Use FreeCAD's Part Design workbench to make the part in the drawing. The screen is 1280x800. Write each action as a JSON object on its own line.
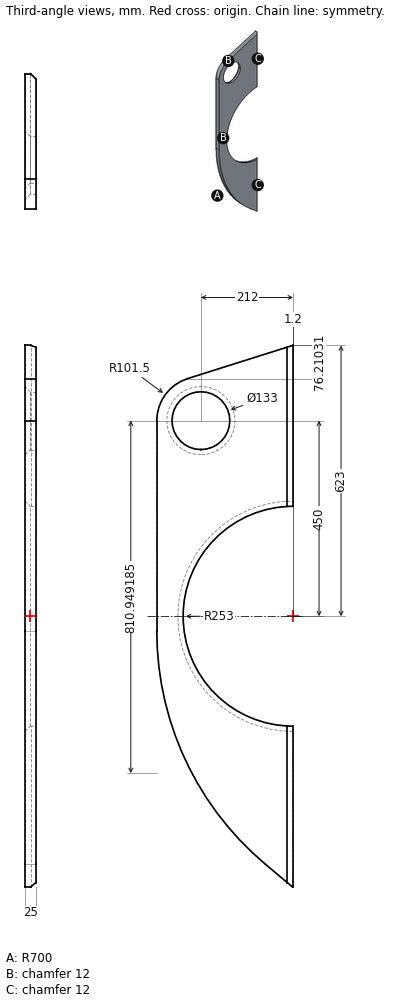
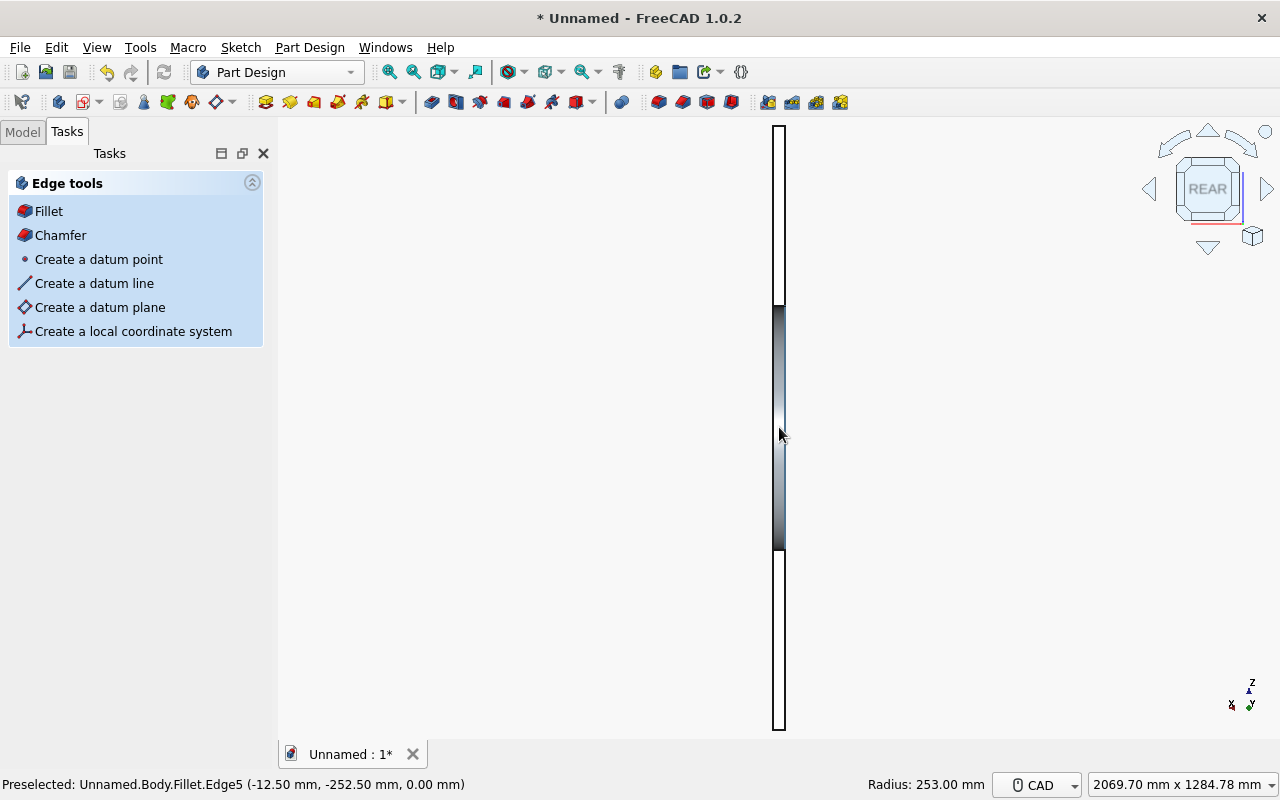
{"action": "key", "text": "6"}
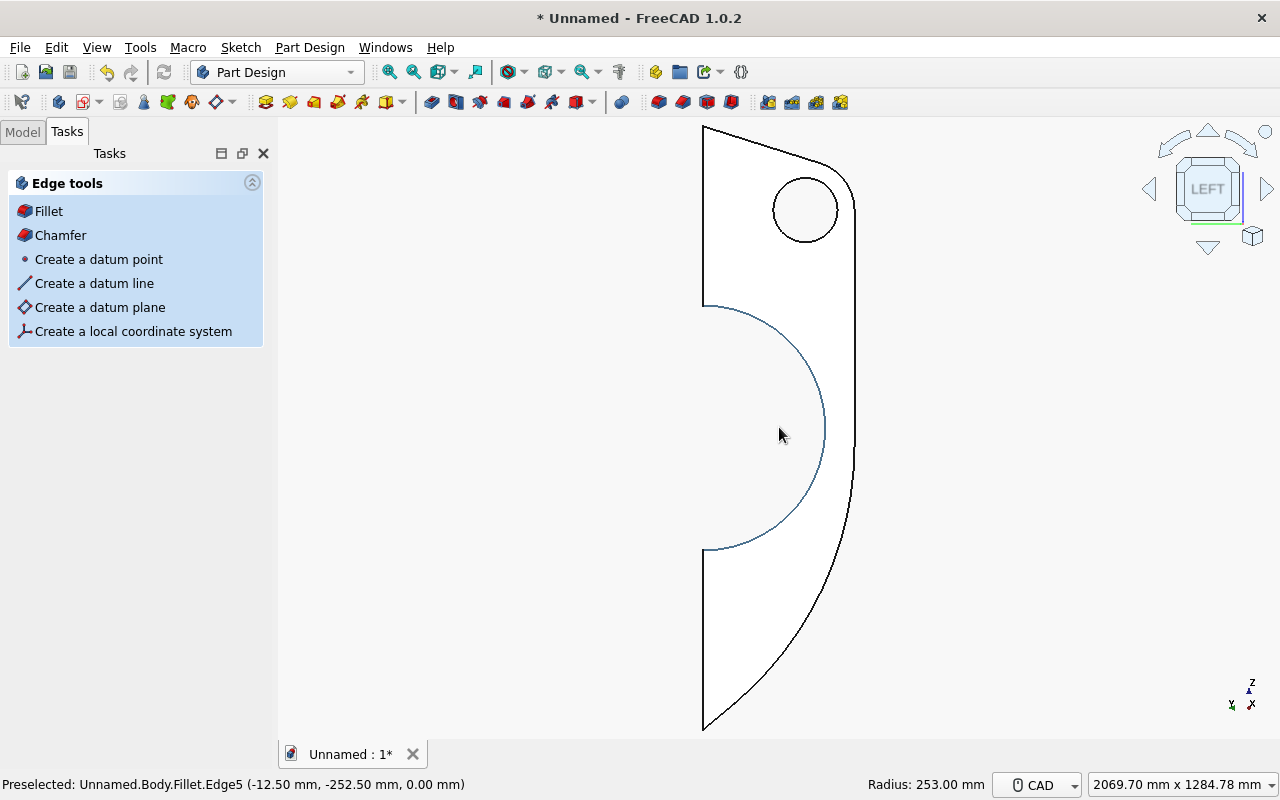
{"action": "left_click", "coordinate": [838, 209], "text": "ctrl"}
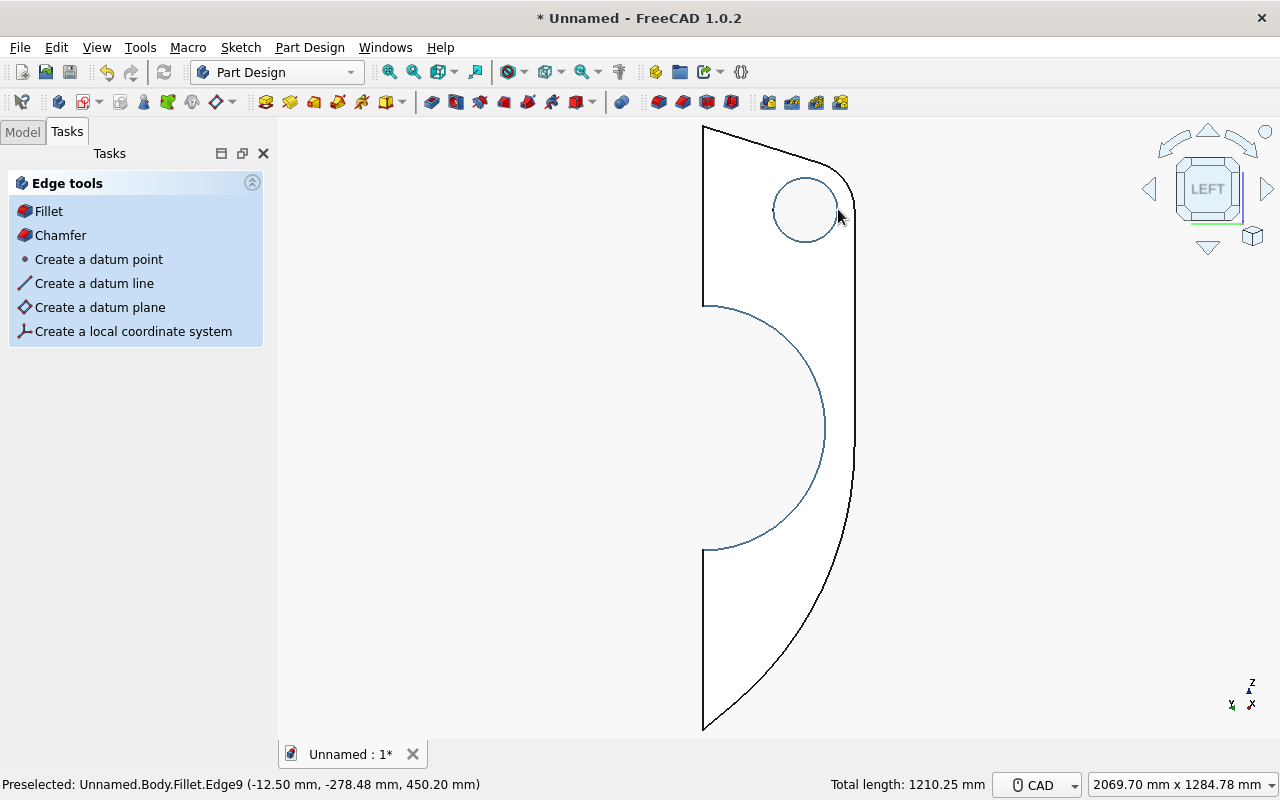
{"action": "left_click", "coordinate": [684, 102]}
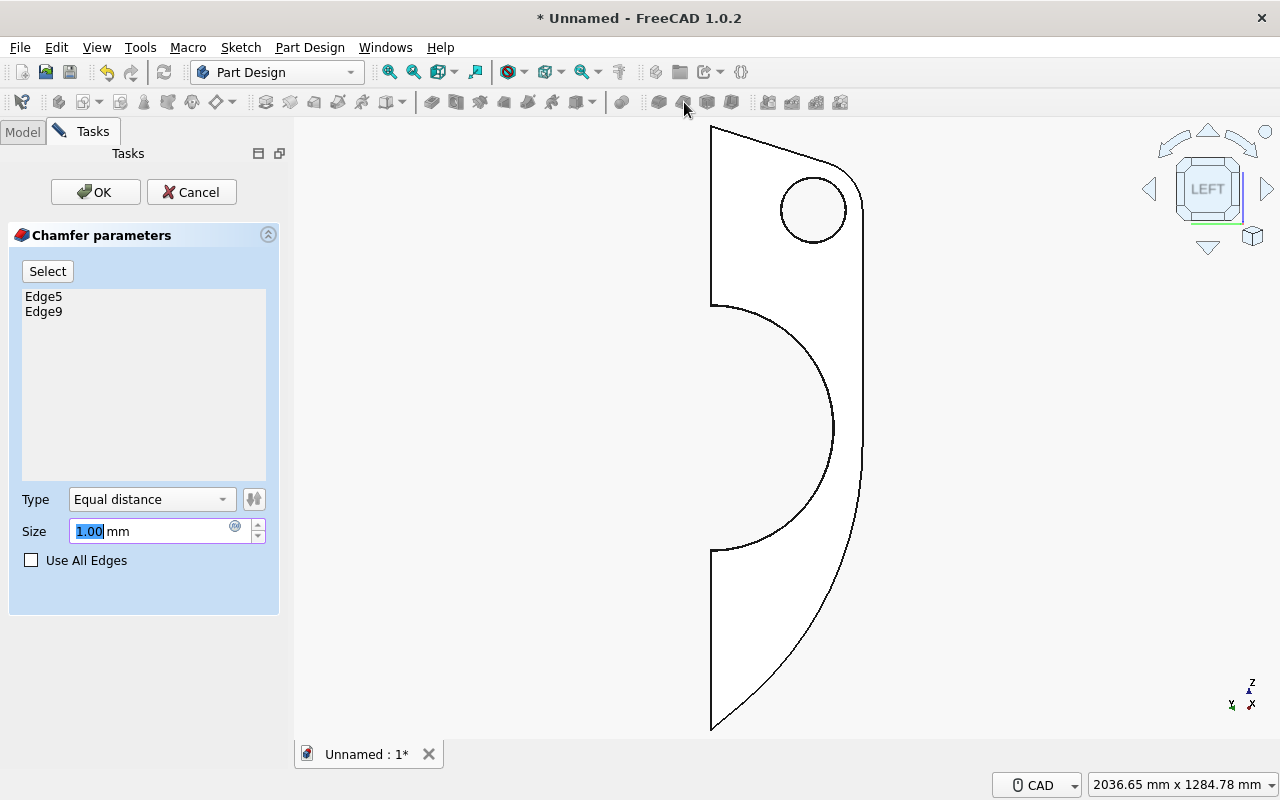
{"action": "type", "text": "12"}
{"action": "key", "text": "Tab"}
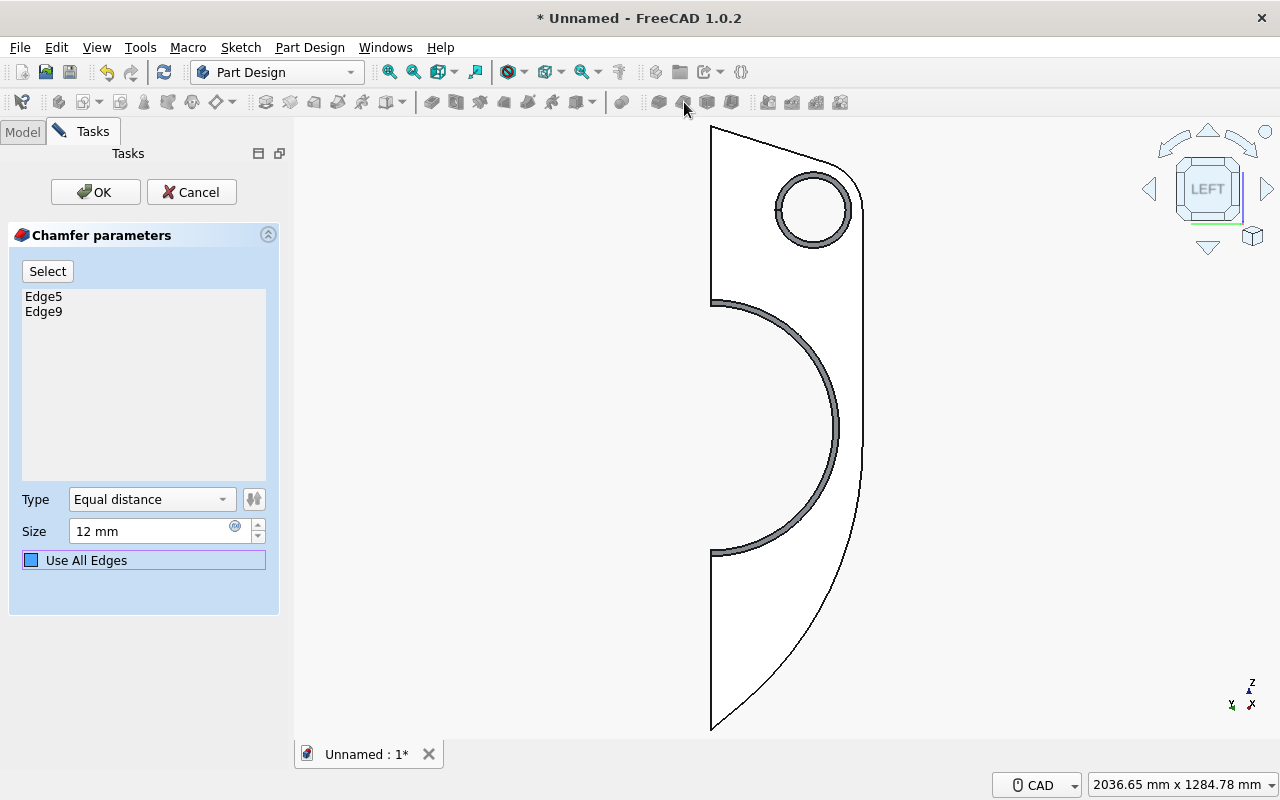
{"action": "left_click", "coordinate": [96, 192]}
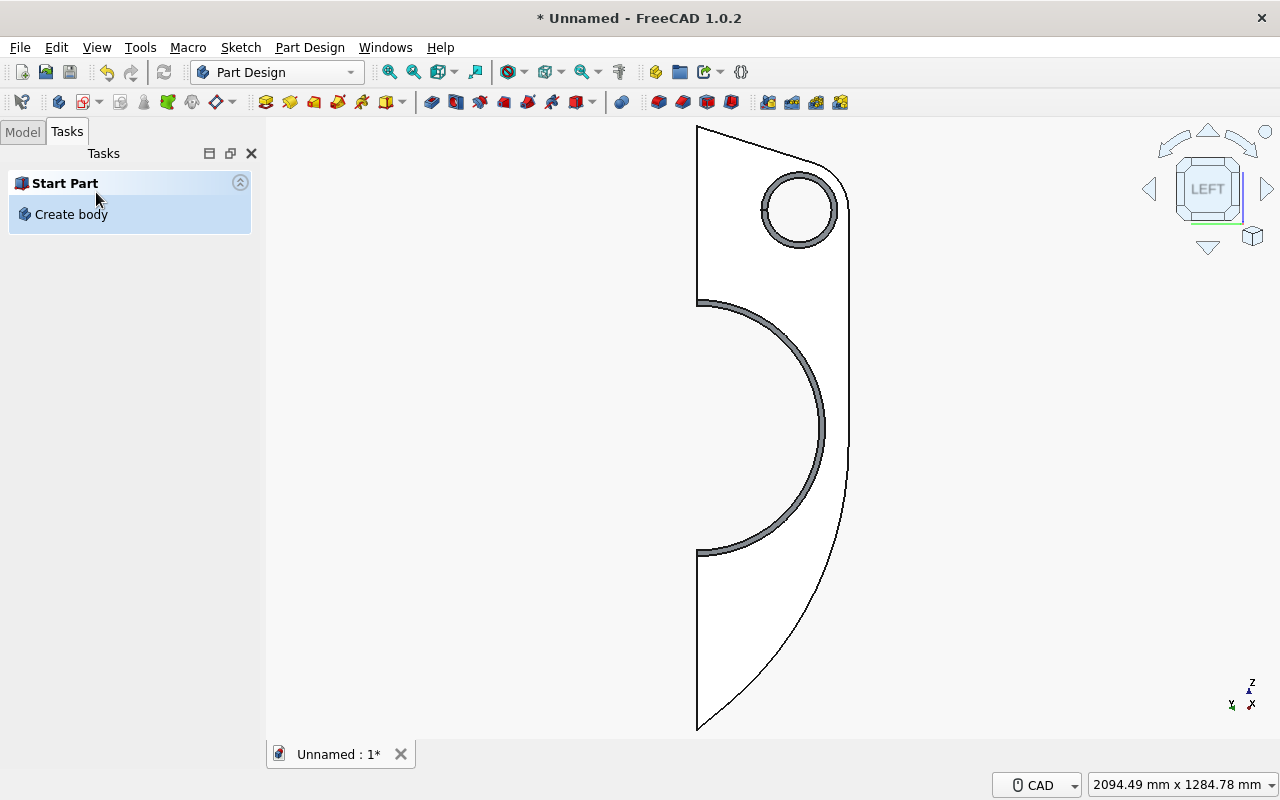
{"action": "key", "text": "0"}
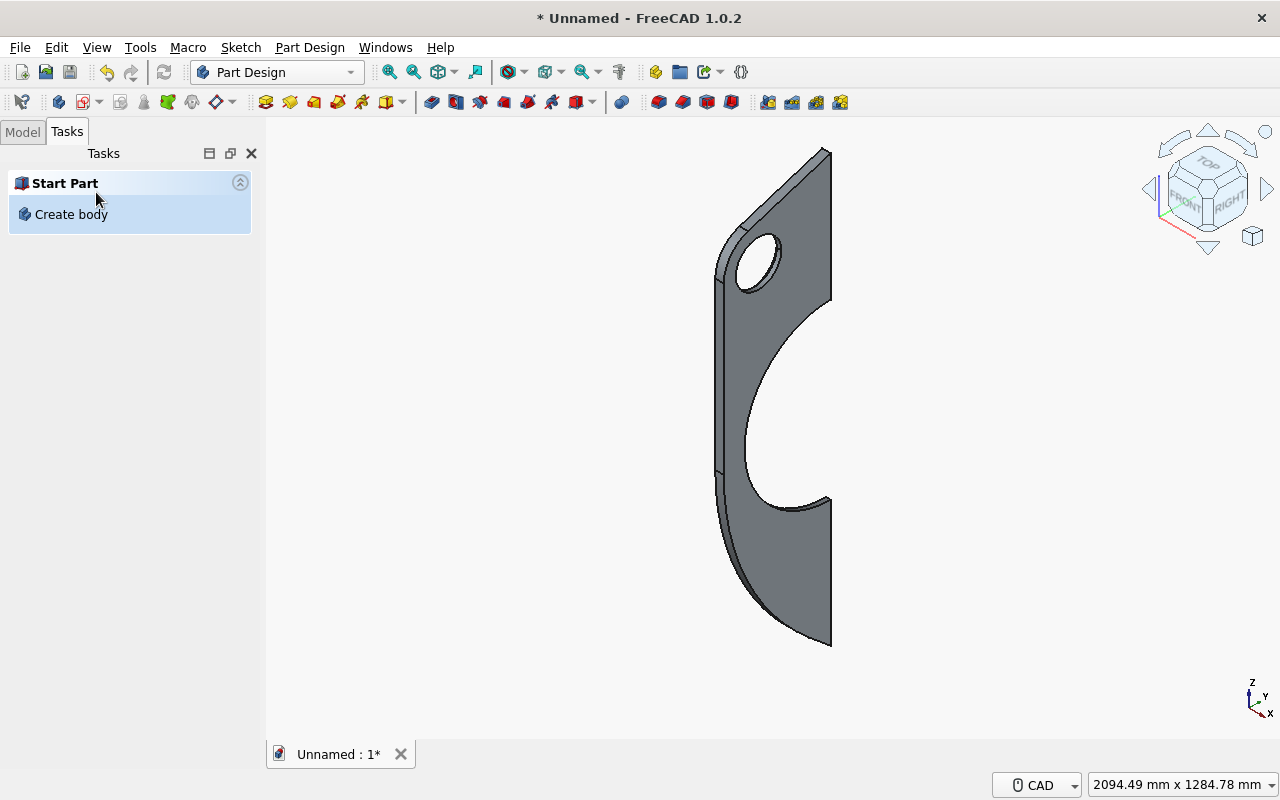
{"action": "key", "text": "2"}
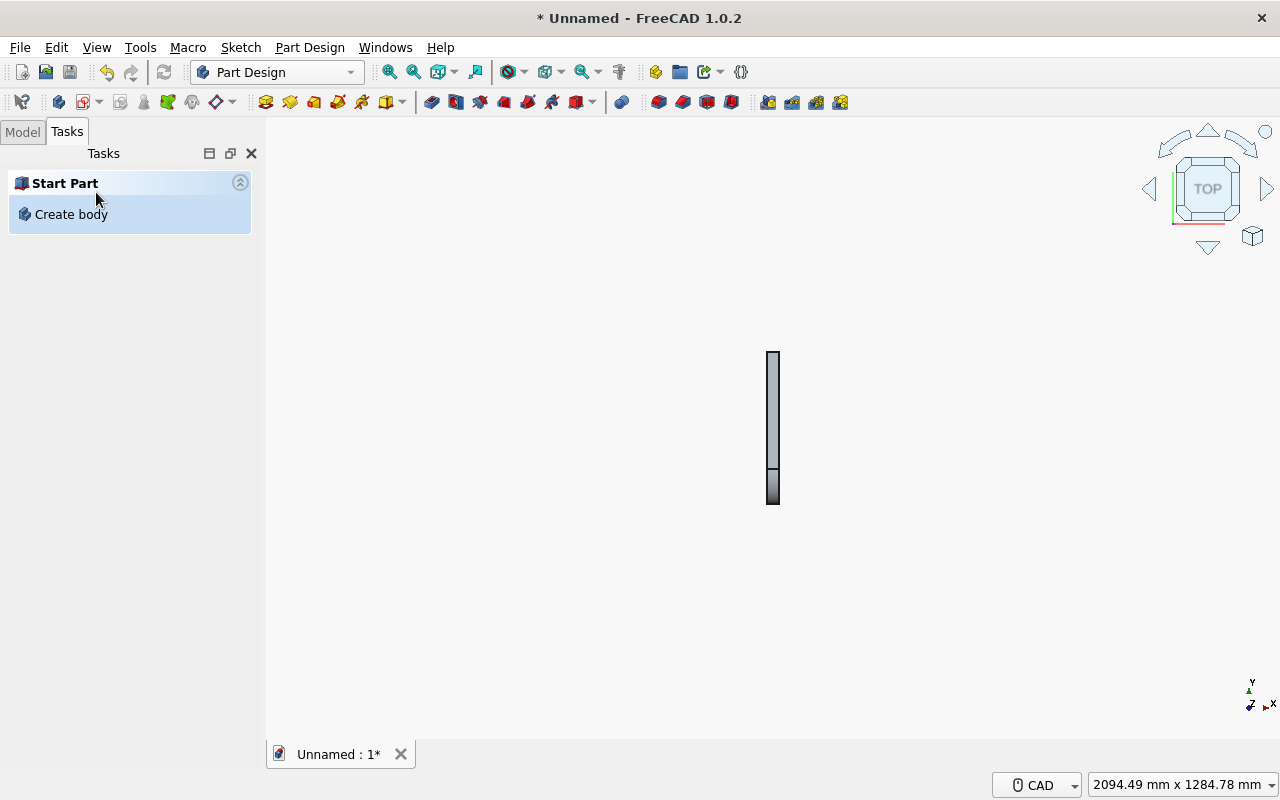
{"action": "left_click", "coordinate": [390, 72]}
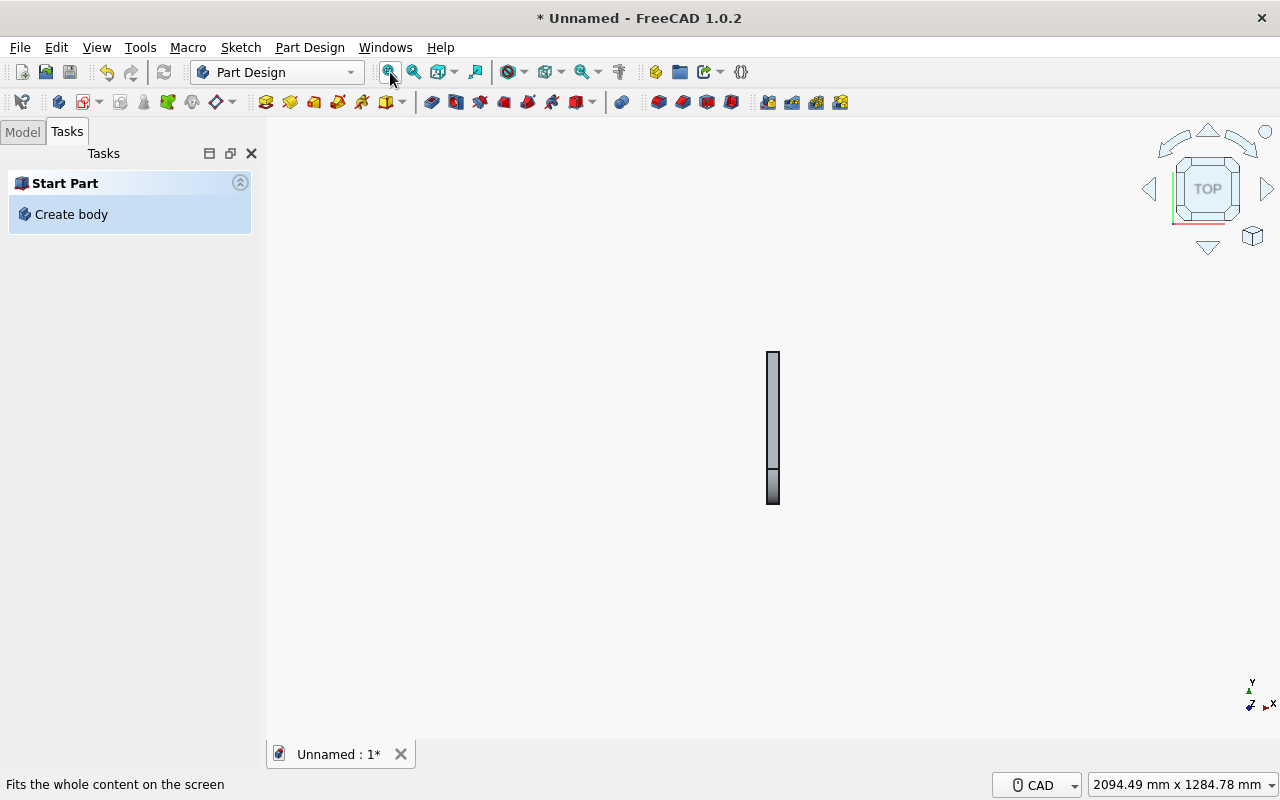
{"action": "key", "text": "1"}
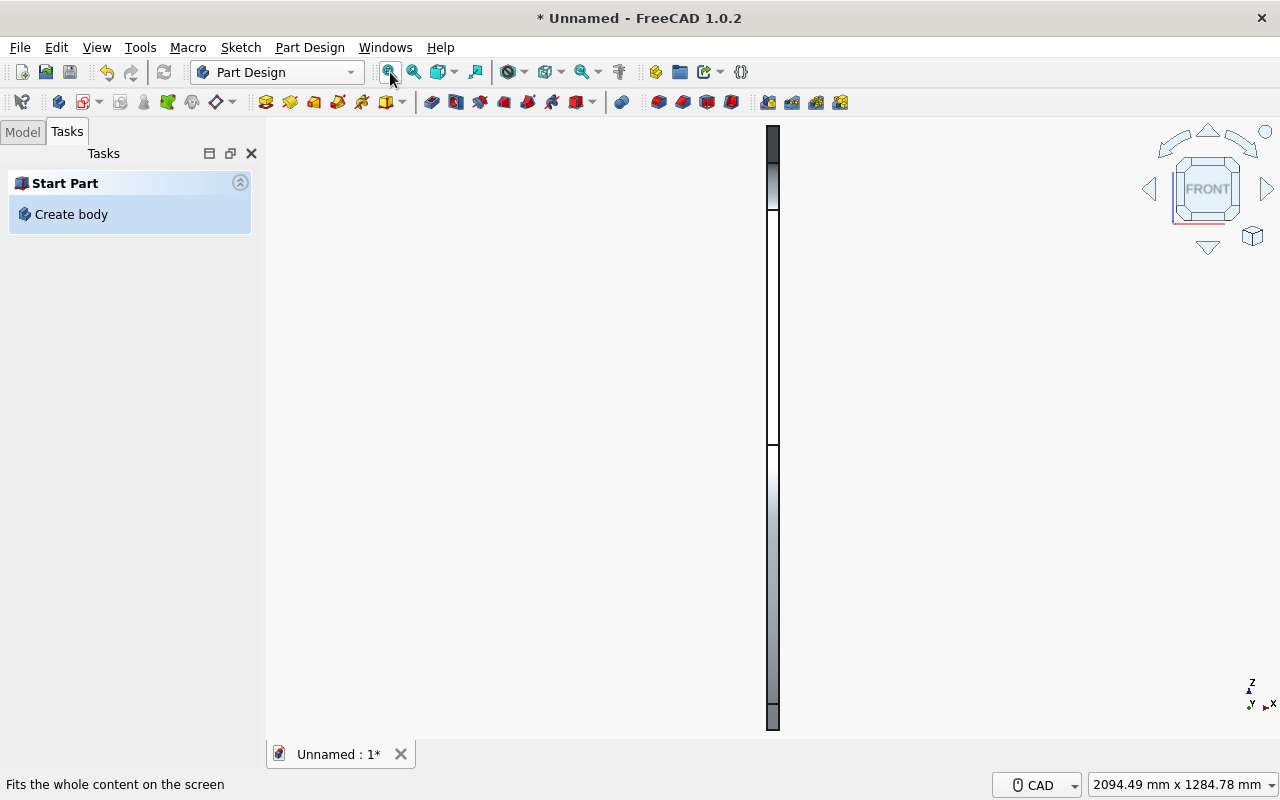
{"action": "key", "text": "3"}